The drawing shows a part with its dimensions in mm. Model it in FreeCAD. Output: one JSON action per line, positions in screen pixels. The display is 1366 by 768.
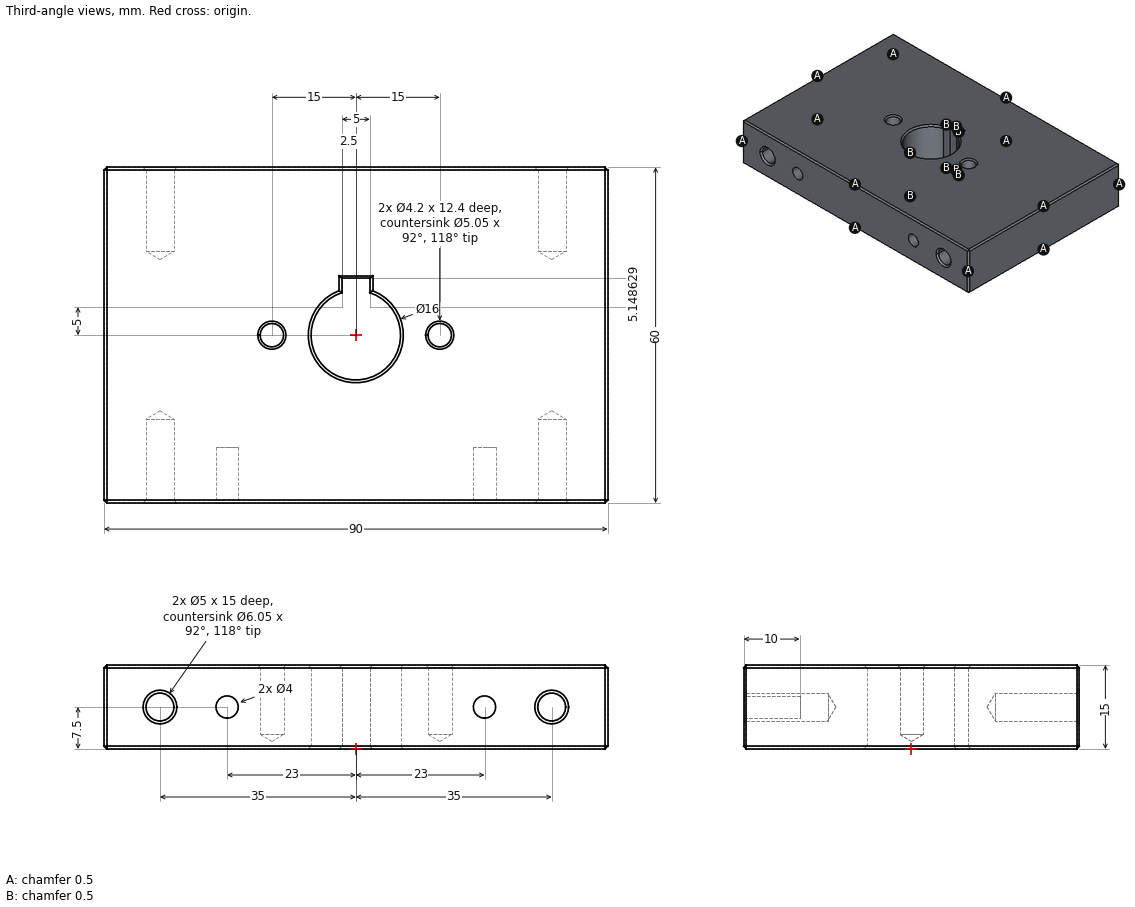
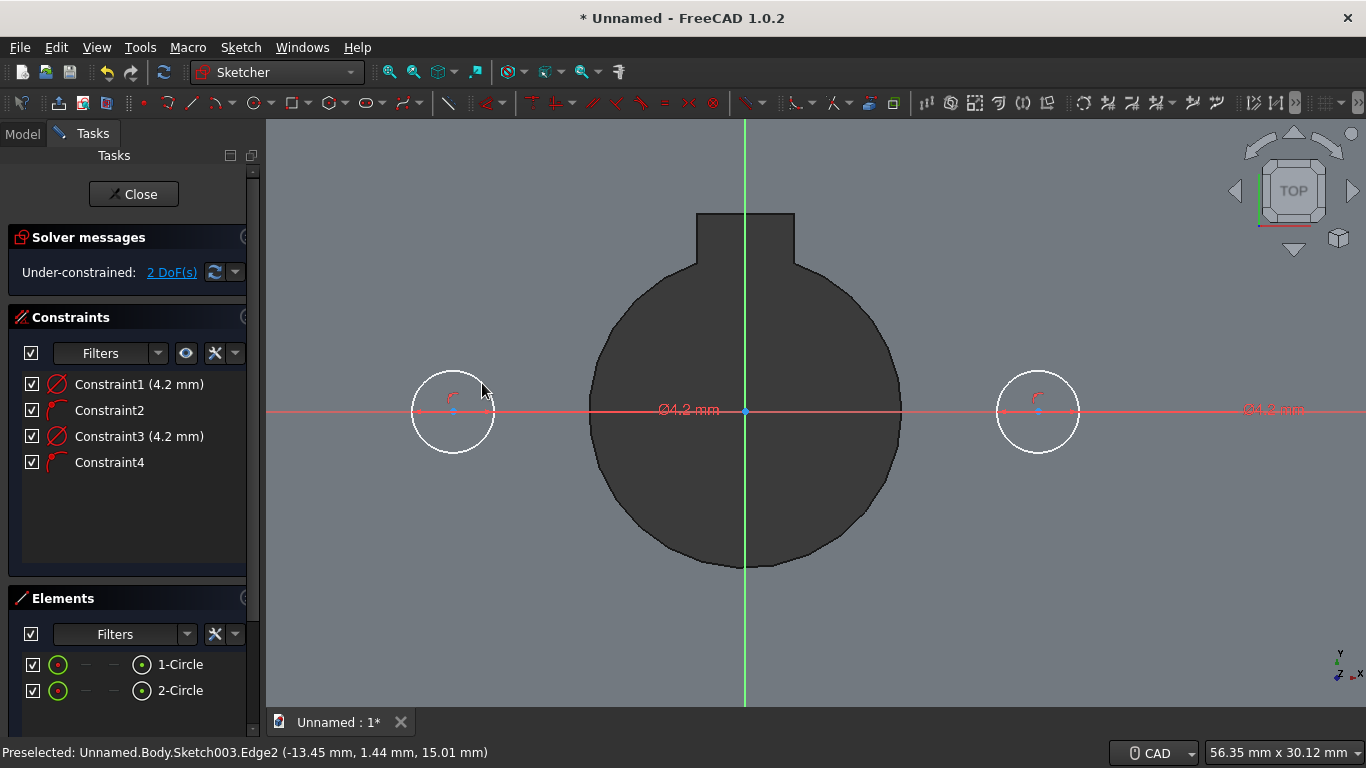
{"action": "key", "text": "d"}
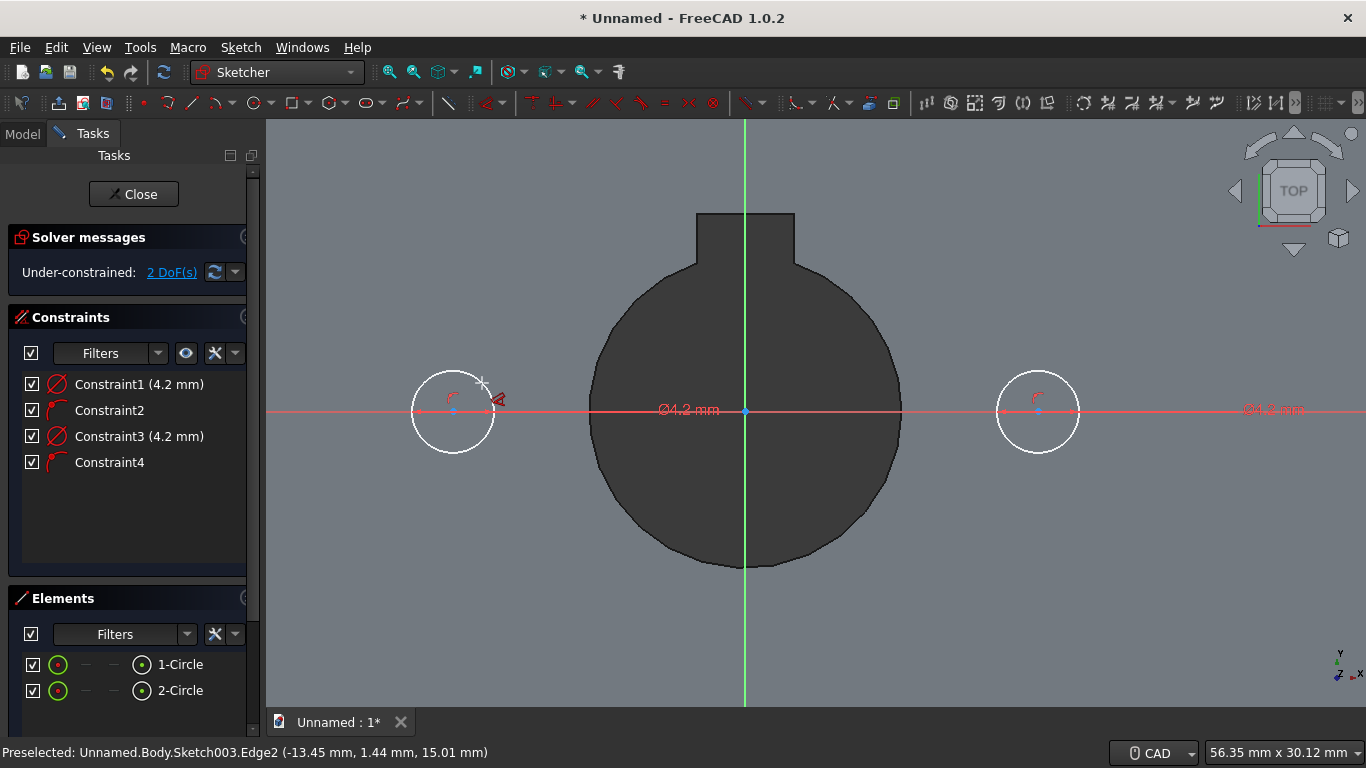
{"action": "left_click", "coordinate": [1038, 412]}
{"action": "left_click", "coordinate": [892, 446]}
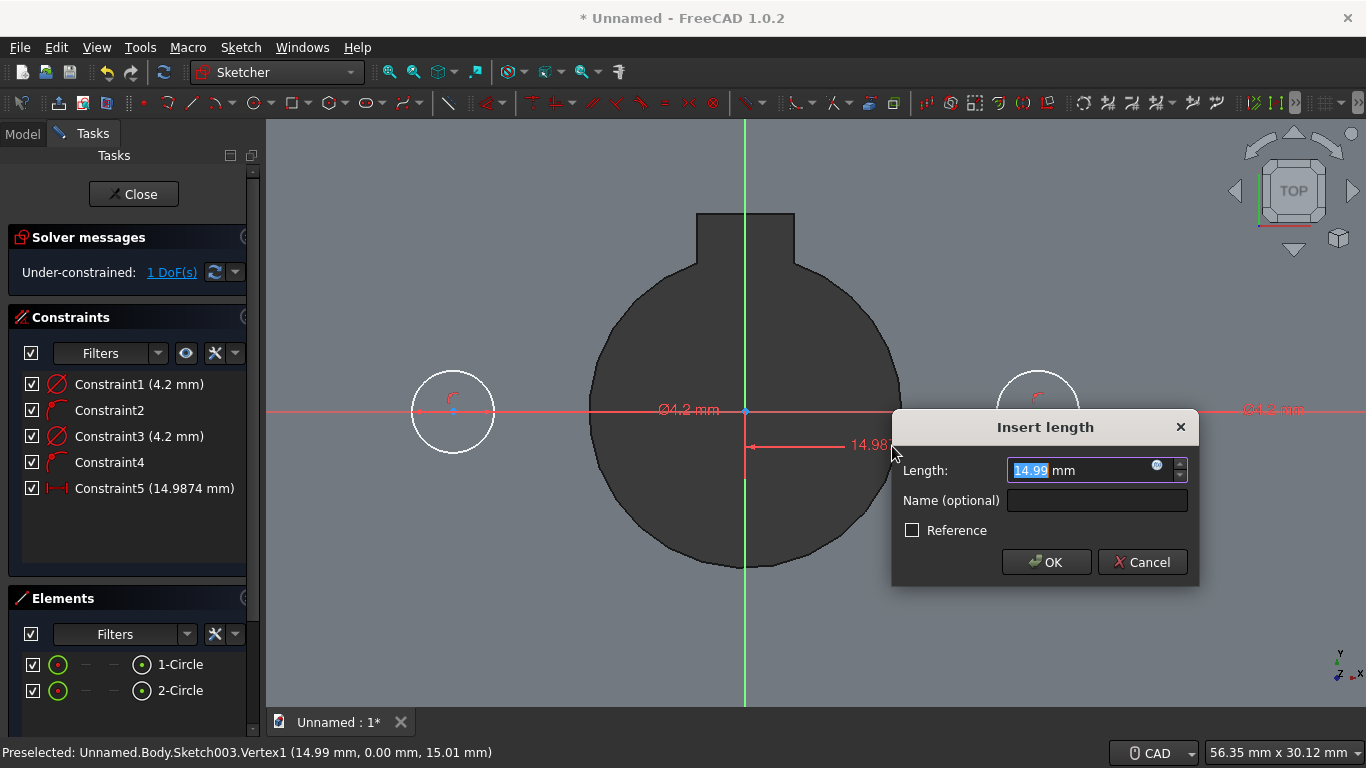
{"action": "type", "text": "15"}
{"action": "key", "text": "Return"}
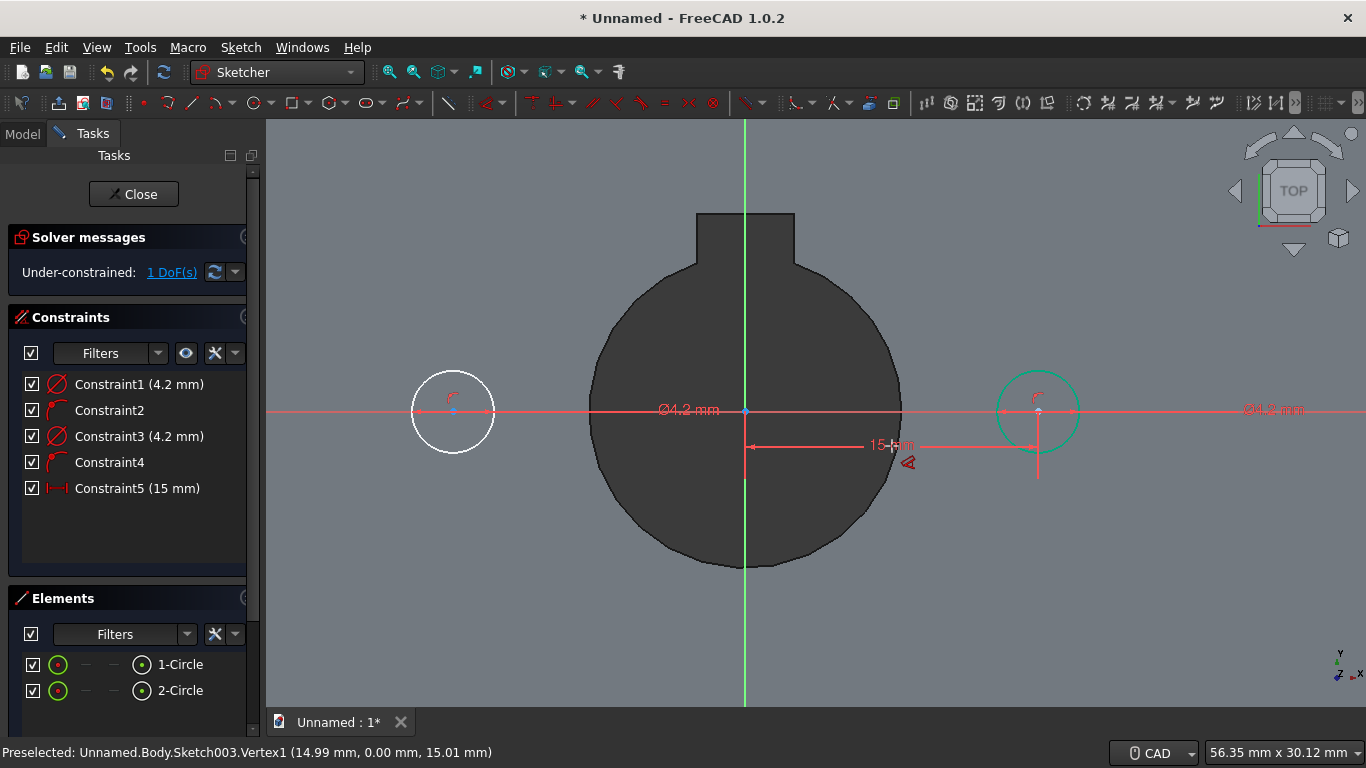
{"action": "left_click", "coordinate": [453, 412]}
{"action": "left_click", "coordinate": [599, 446]}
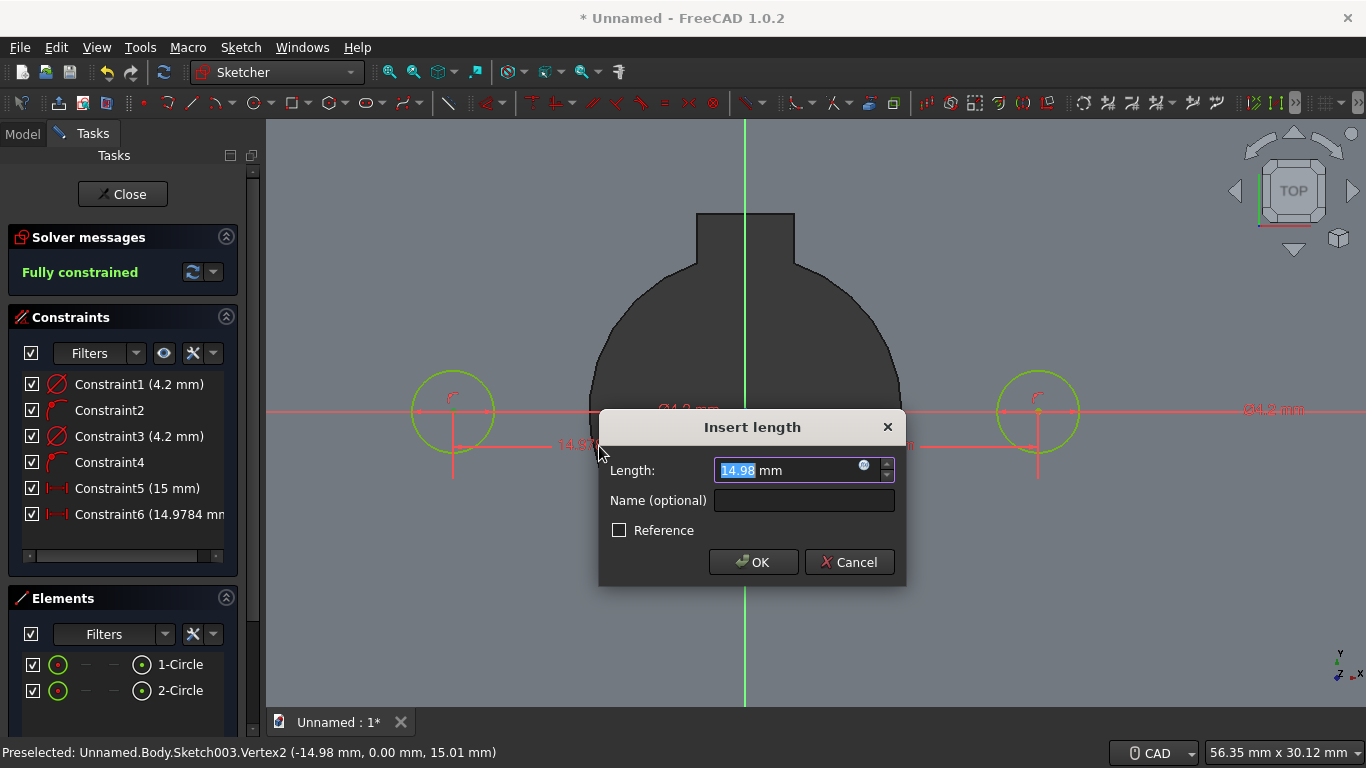
{"action": "type", "text": "15"}
{"action": "key", "text": "Return"}
{"action": "key", "text": "Escape"}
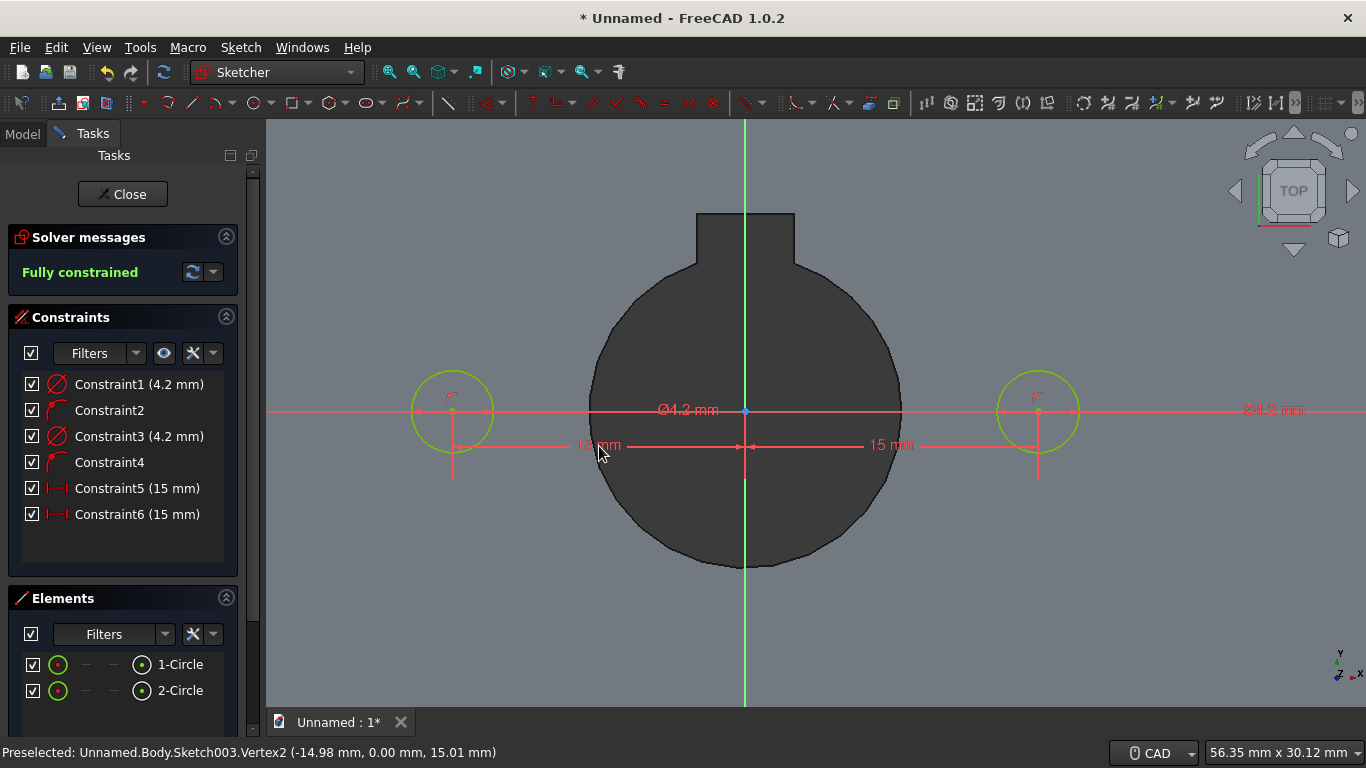
{"action": "left_click", "coordinate": [123, 194]}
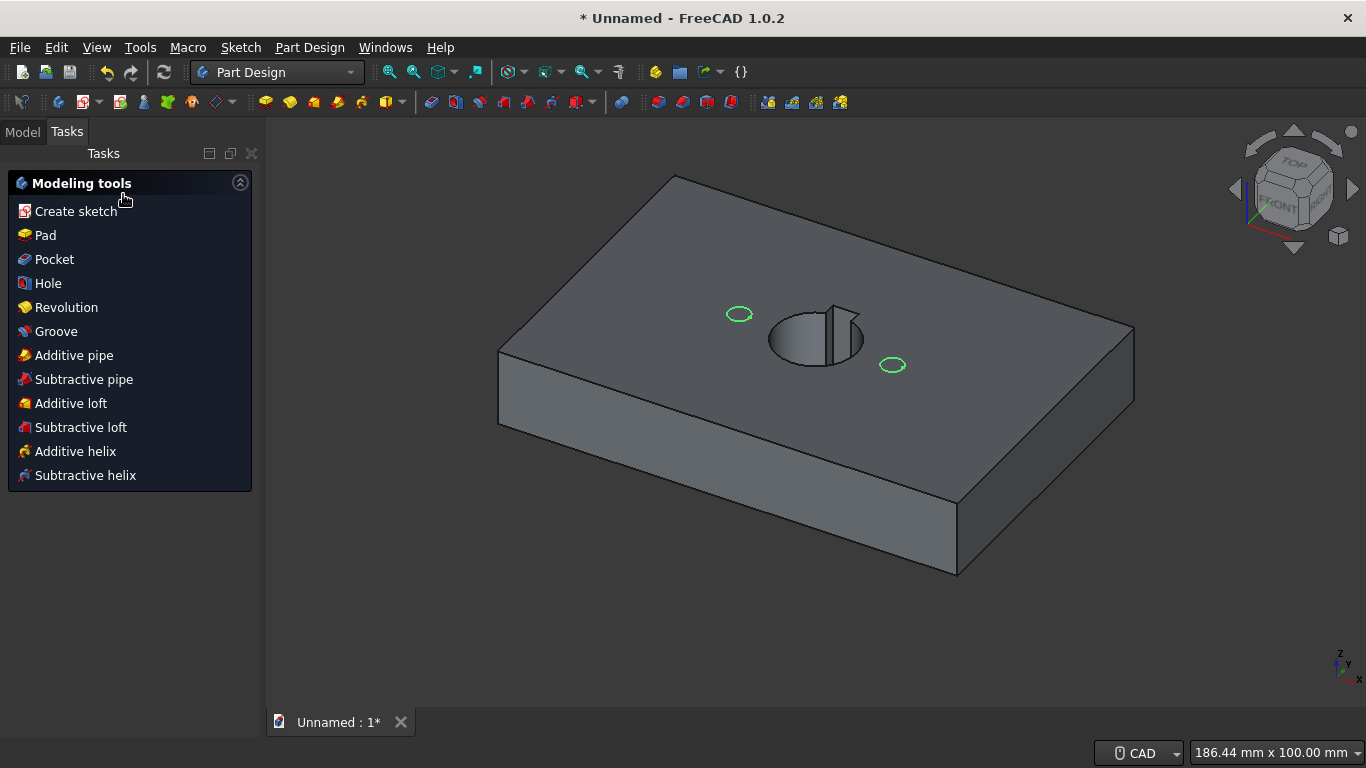
{"action": "left_click", "coordinate": [456, 102]}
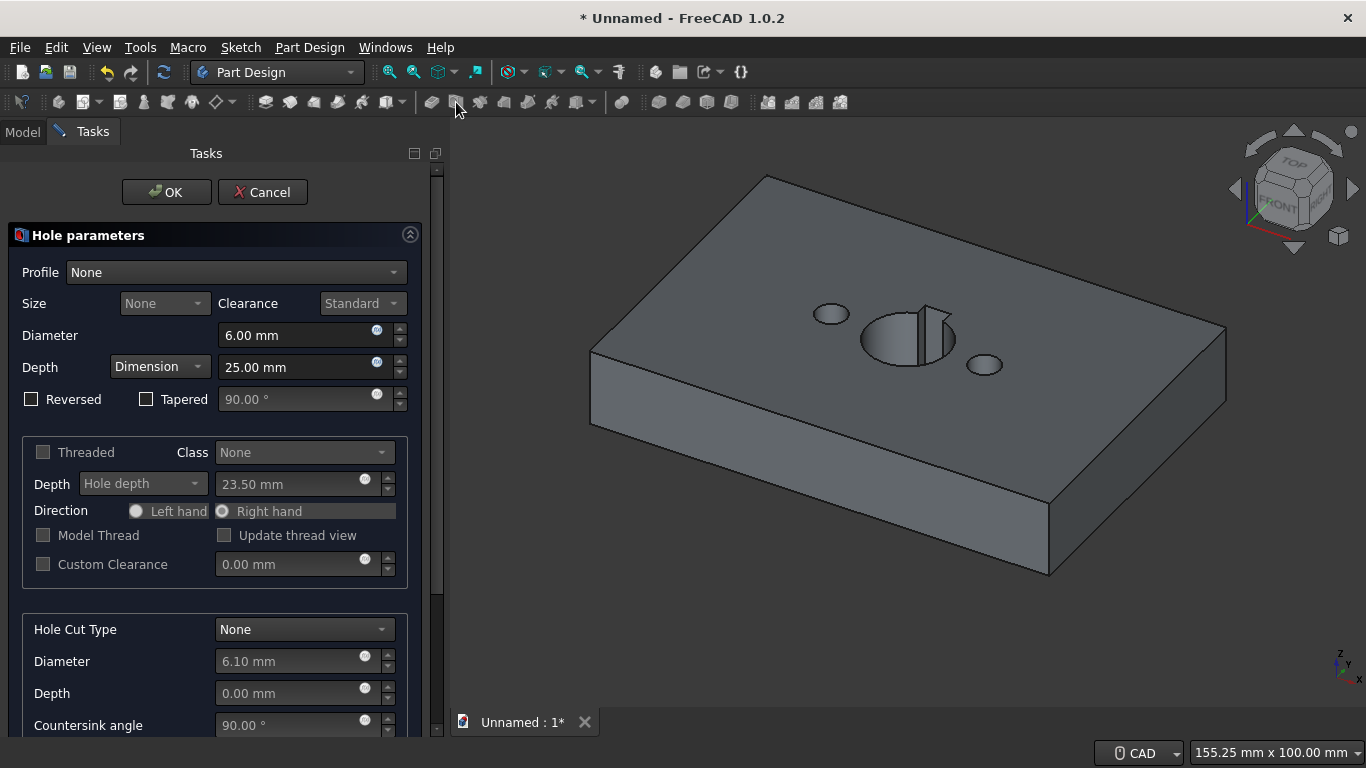
{"action": "triple_click", "coordinate": [305, 335]}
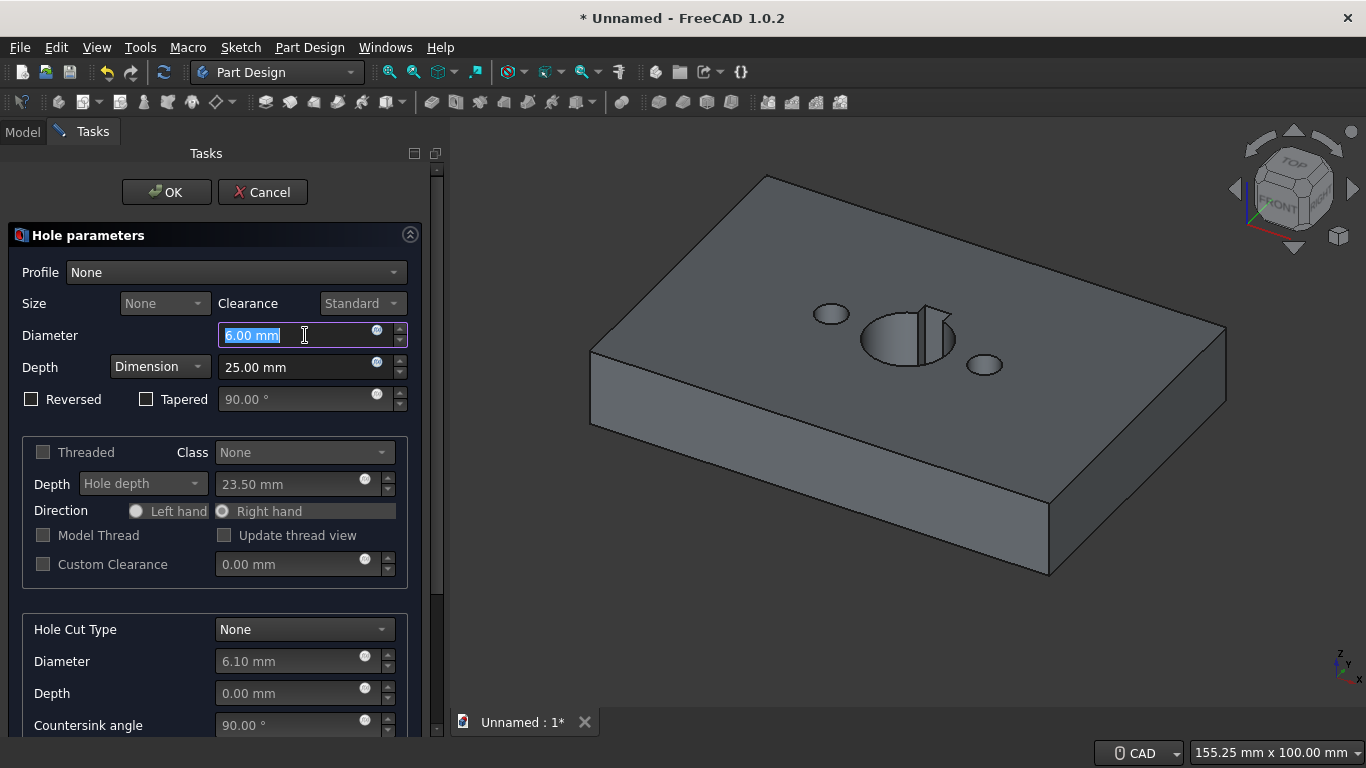
{"action": "type", "text": "4.2"}
{"action": "key", "text": "Tab"}